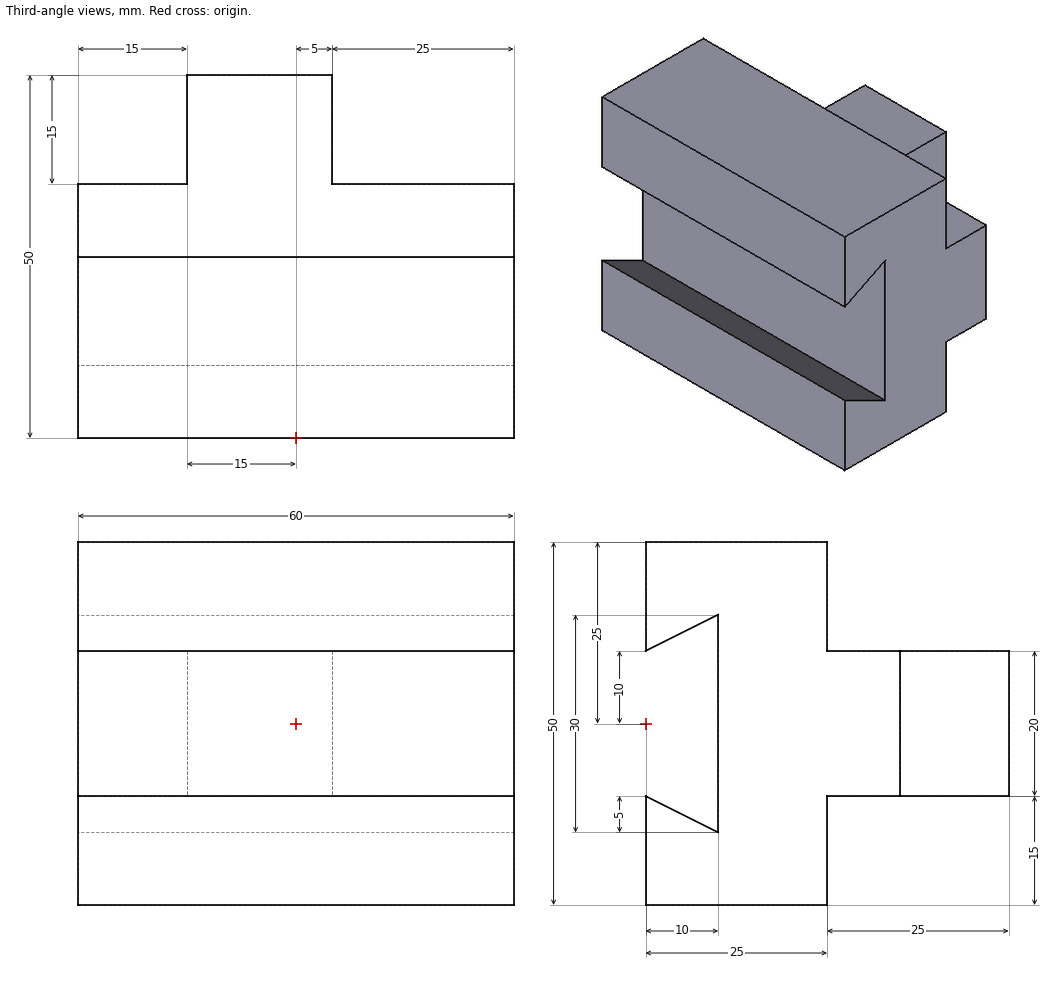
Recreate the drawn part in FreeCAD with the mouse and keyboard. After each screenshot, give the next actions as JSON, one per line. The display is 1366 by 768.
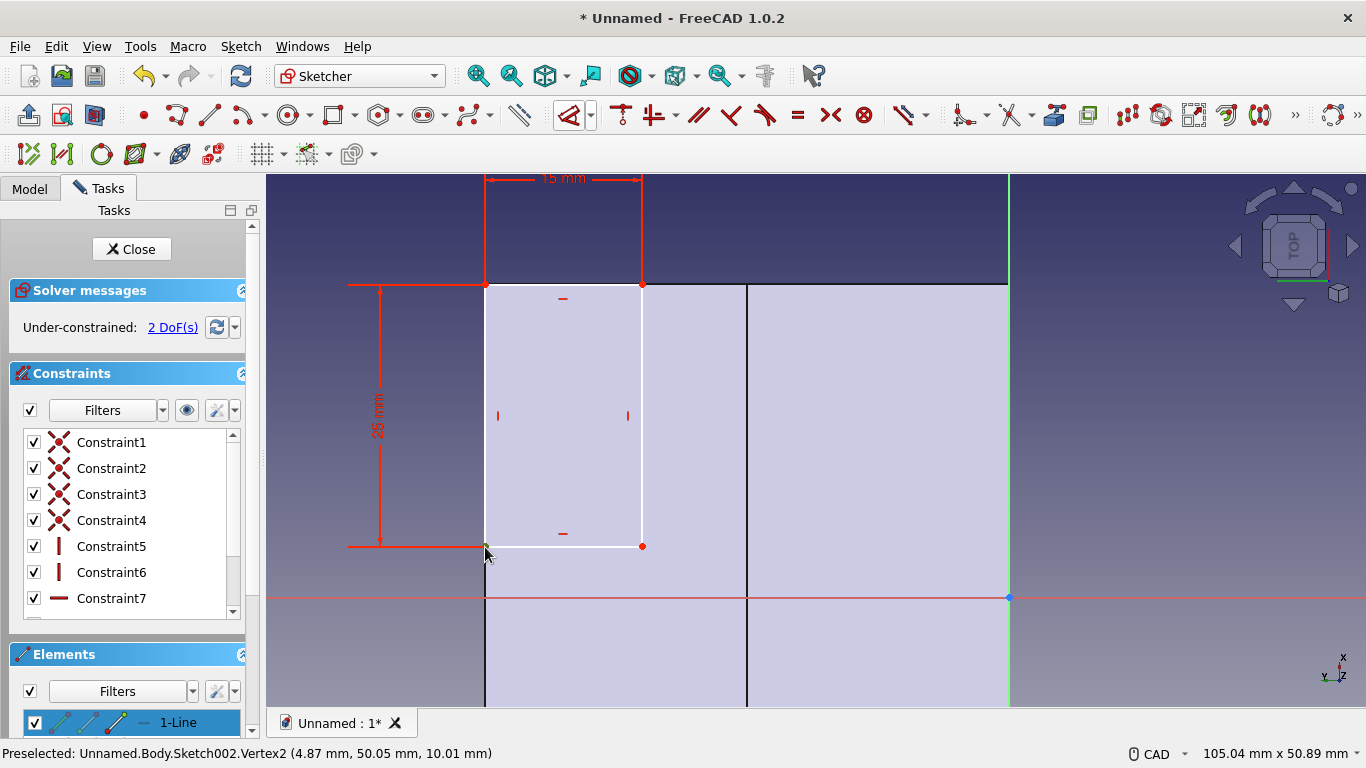
{"action": "key", "text": "i"}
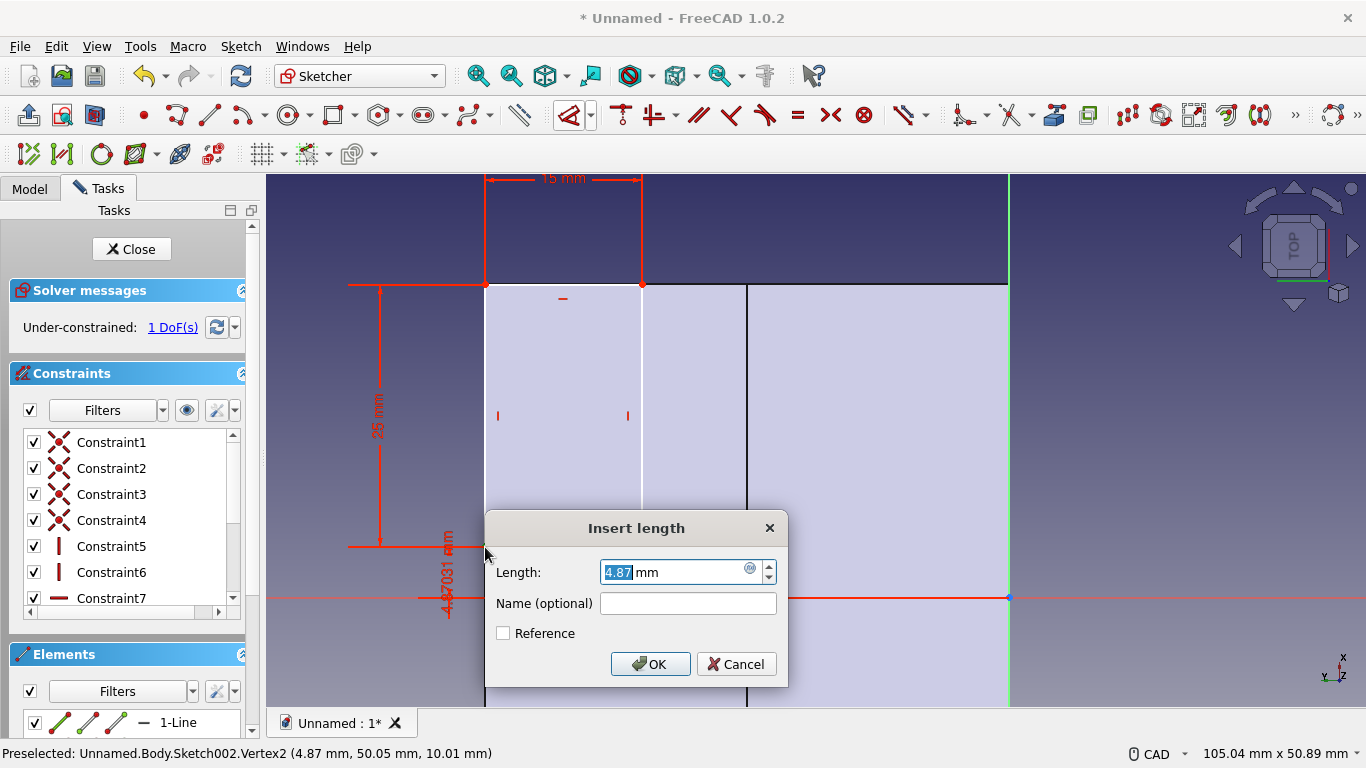
{"action": "type", "text": "5"}
{"action": "key", "text": "Return"}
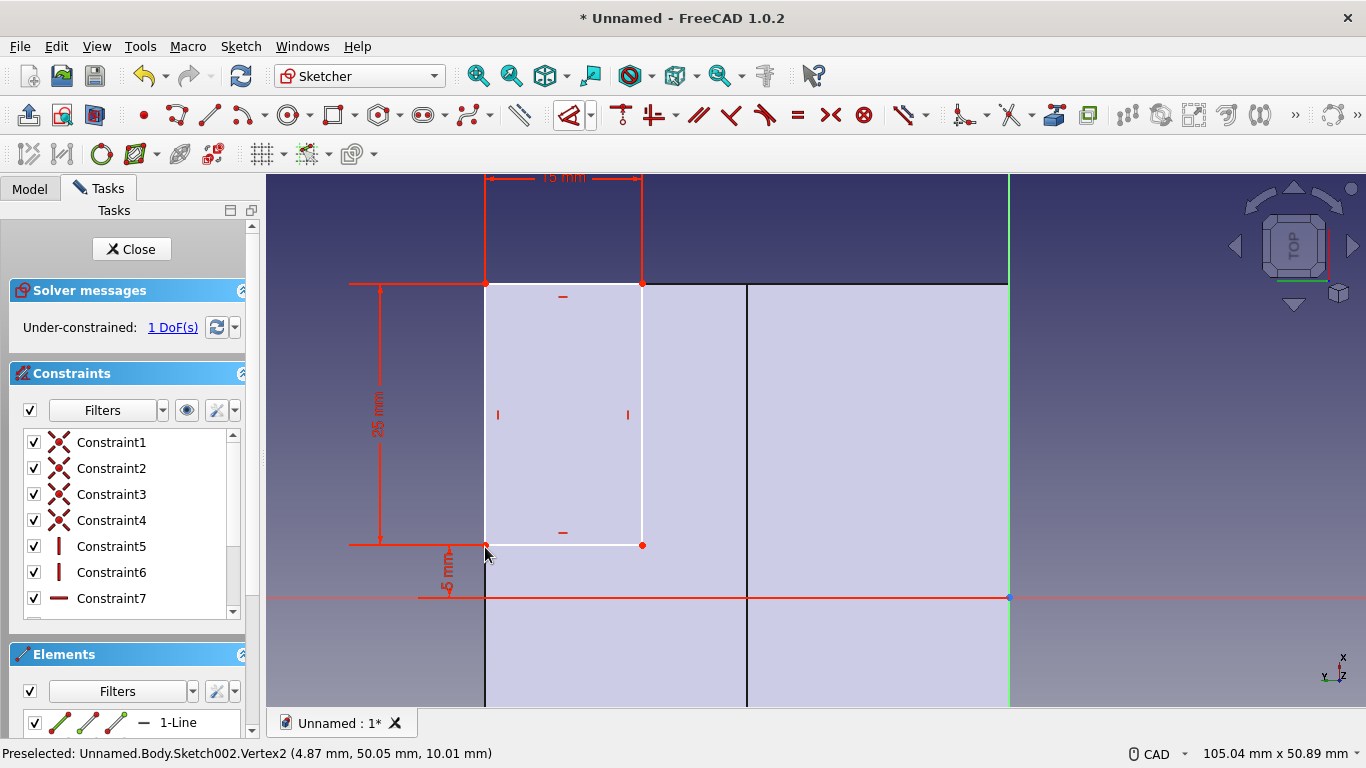
{"action": "left_click", "coordinate": [485, 284]}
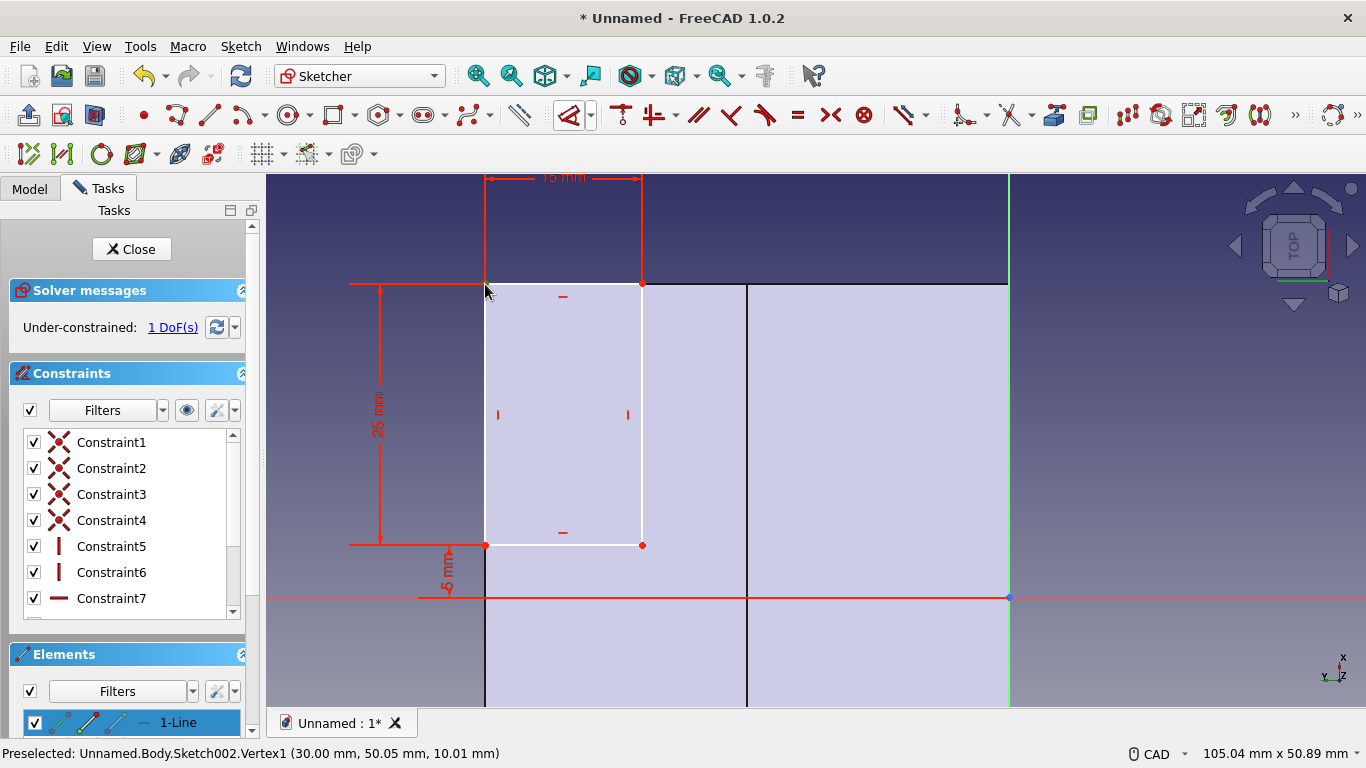
{"action": "key", "text": "l"}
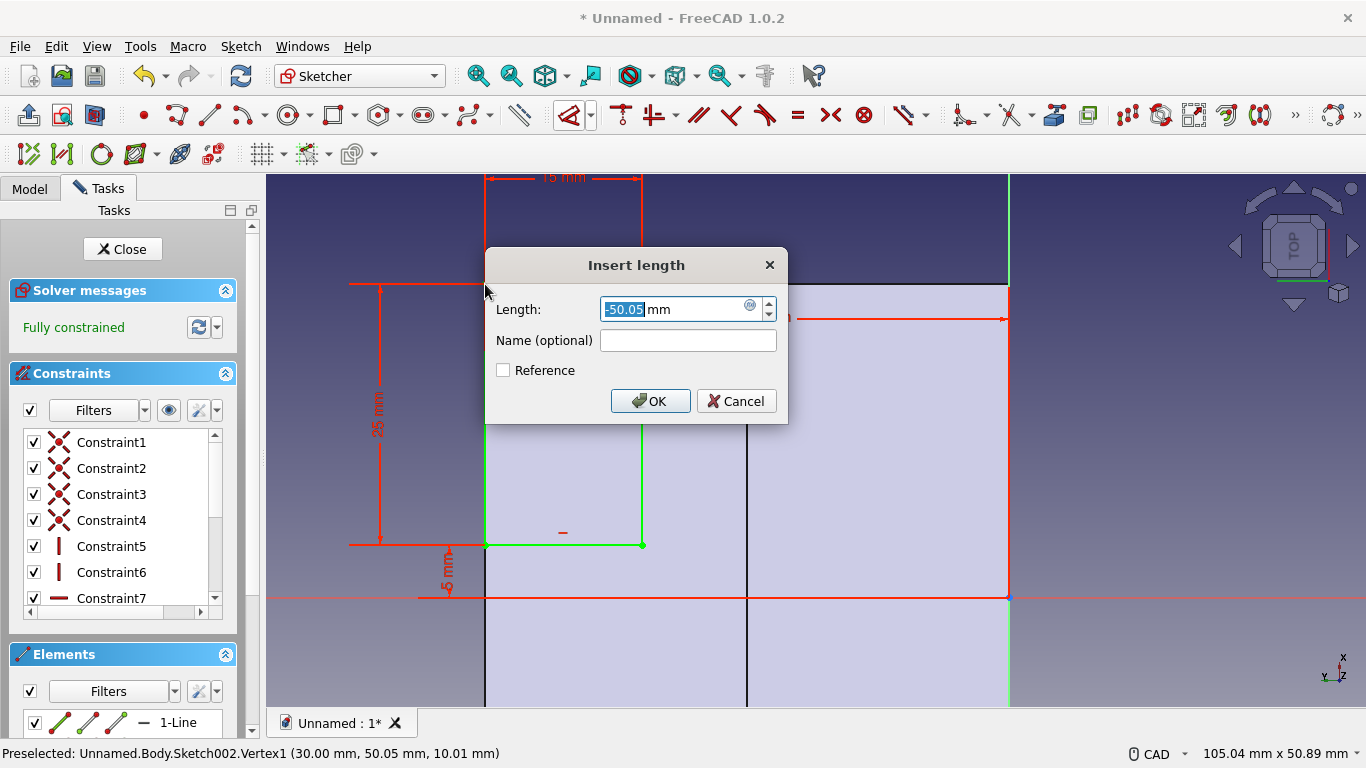
{"action": "type", "text": "-50"}
{"action": "key", "text": "Return"}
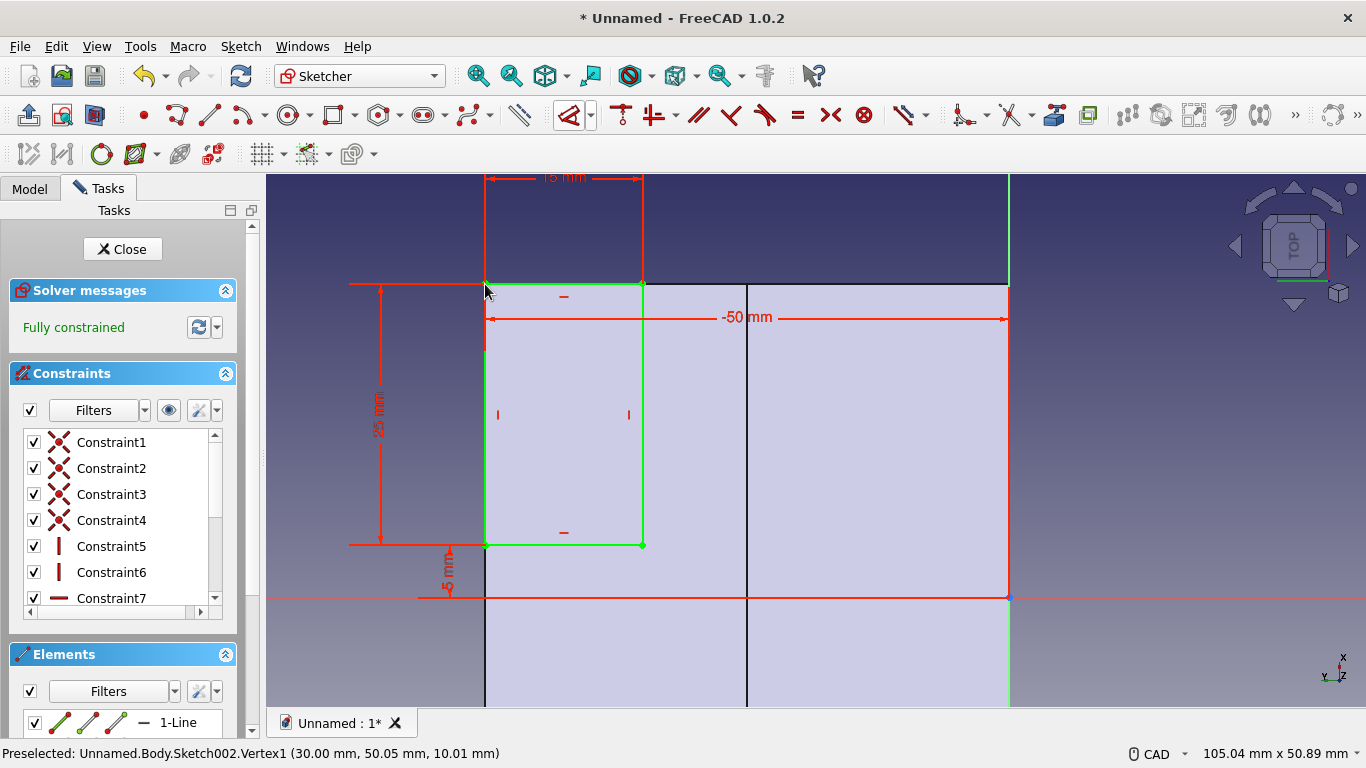
{"action": "left_click", "coordinate": [123, 249]}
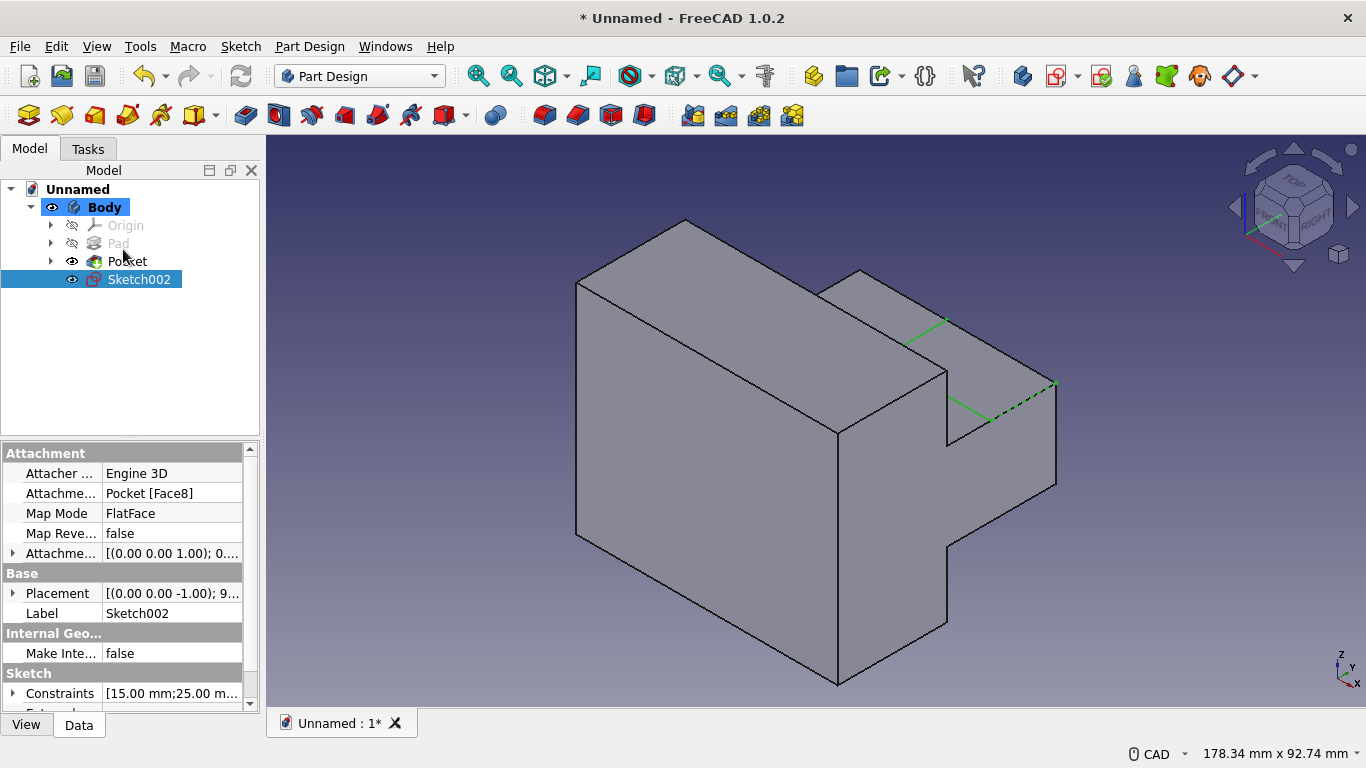
{"action": "left_click", "coordinate": [246, 116]}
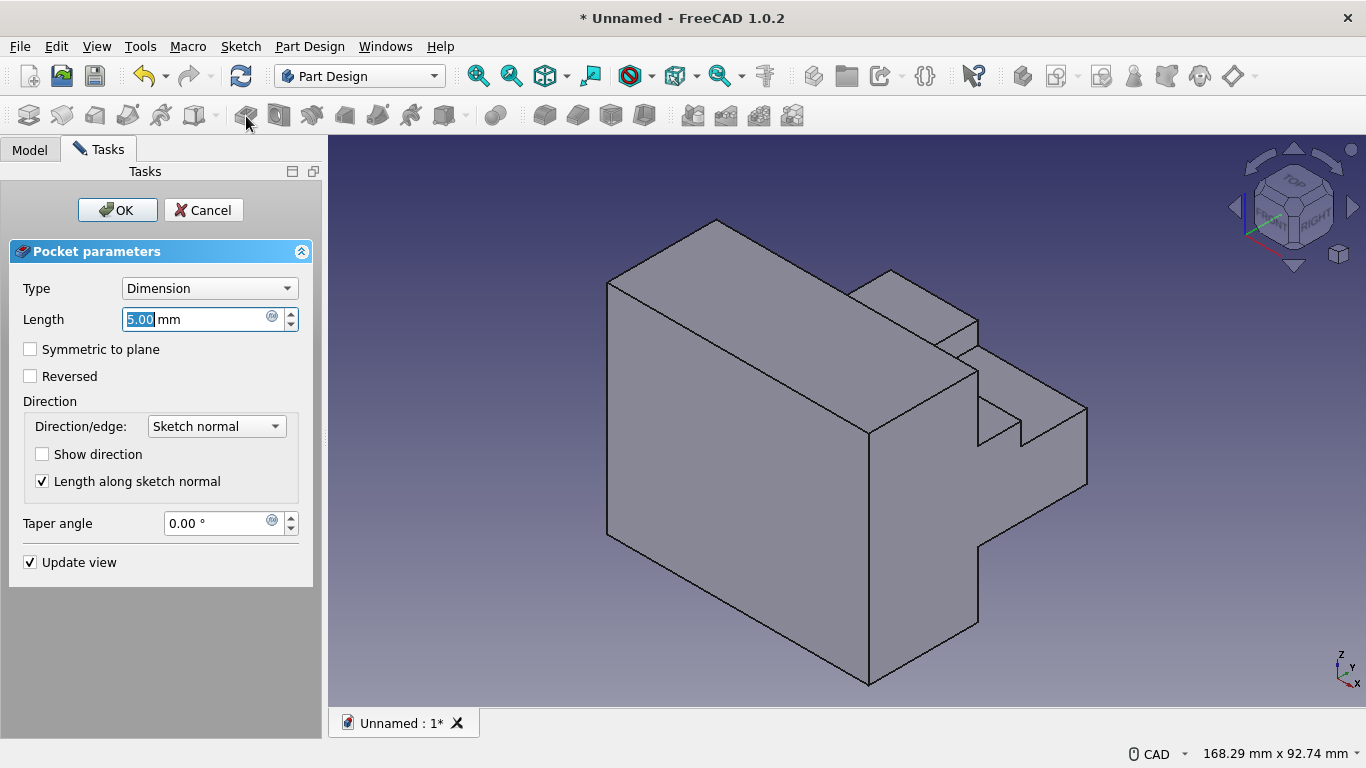
{"action": "left_click", "coordinate": [210, 288]}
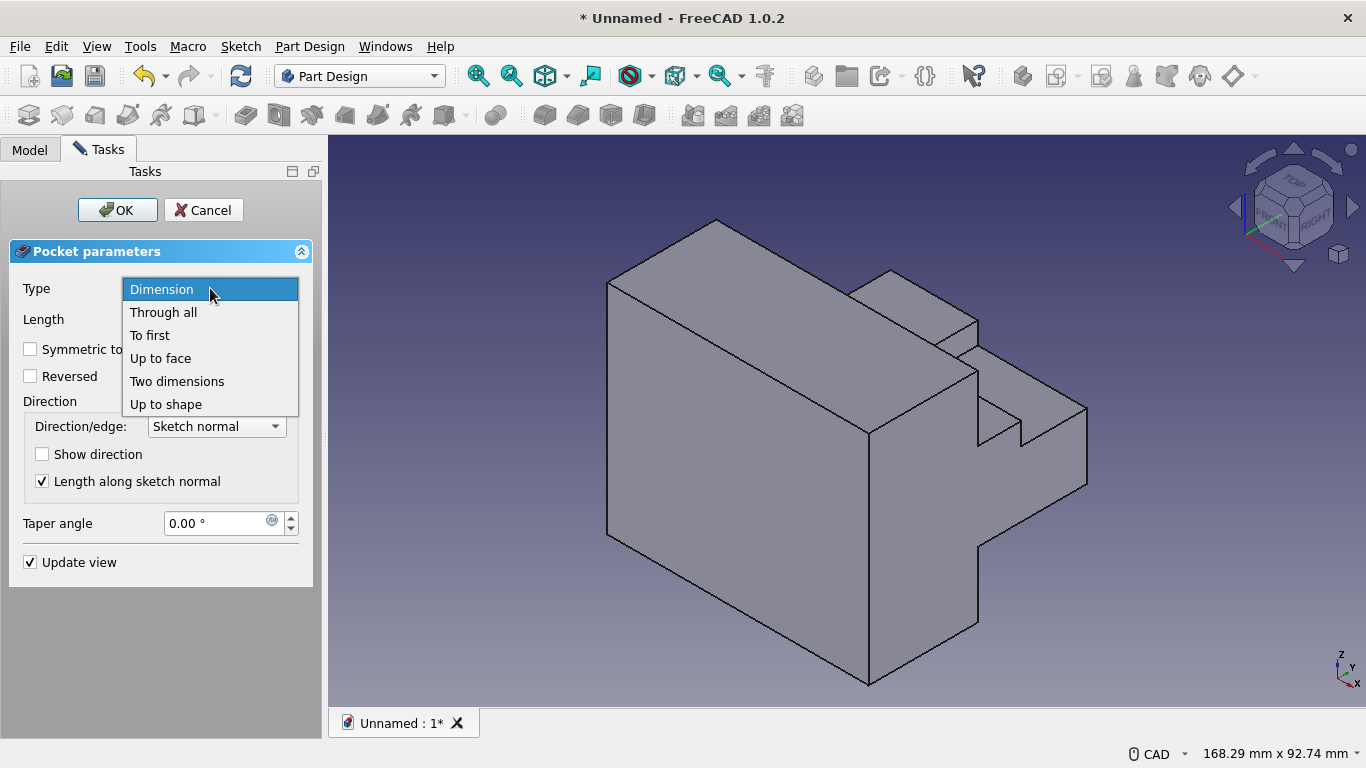
{"action": "left_click", "coordinate": [208, 336]}